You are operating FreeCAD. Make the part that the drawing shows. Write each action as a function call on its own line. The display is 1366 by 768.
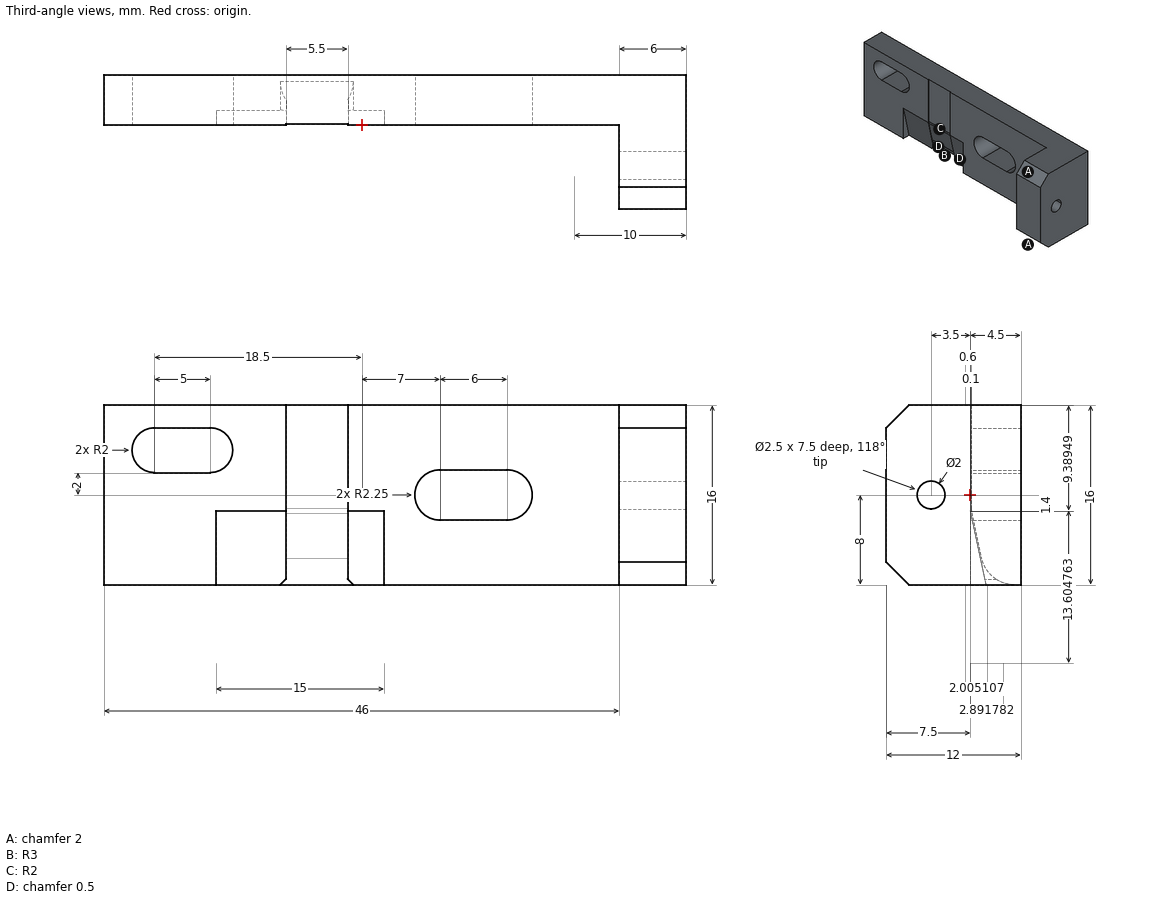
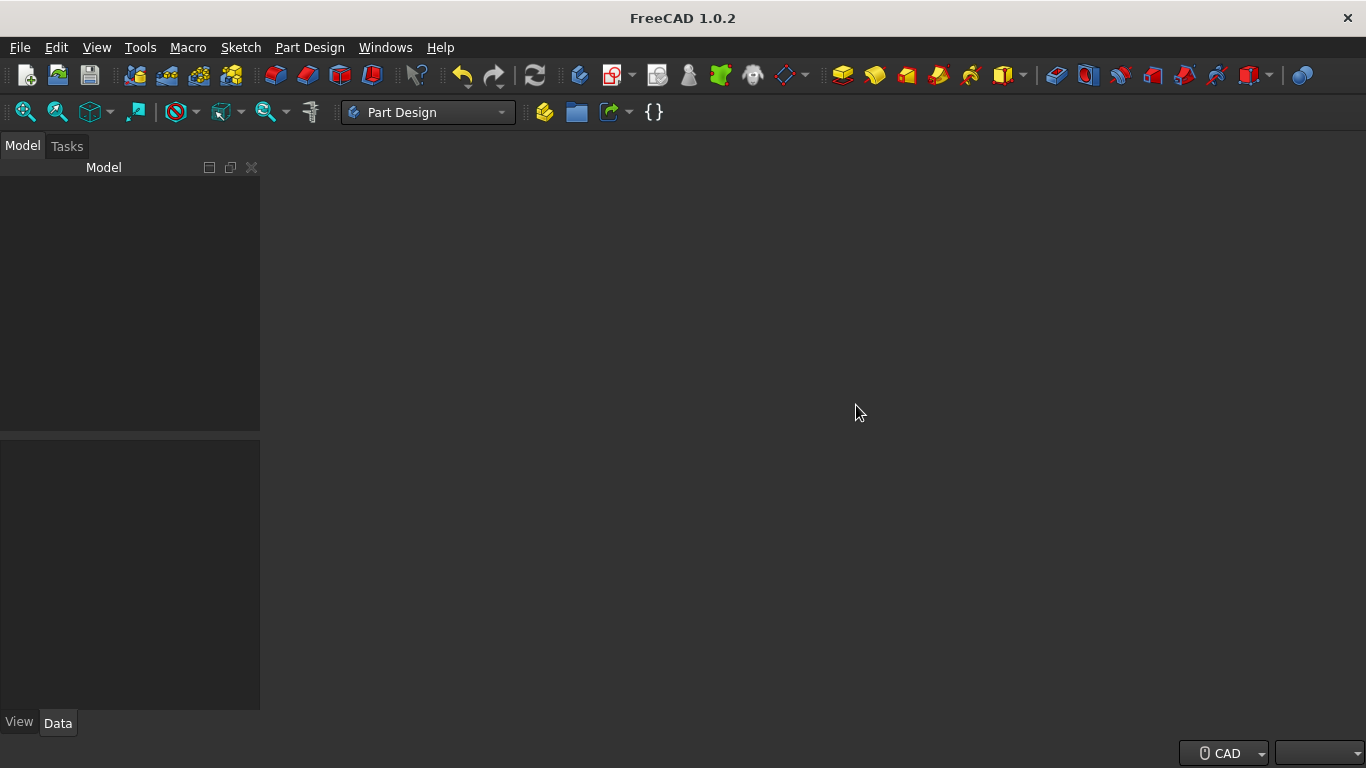
click(26, 76)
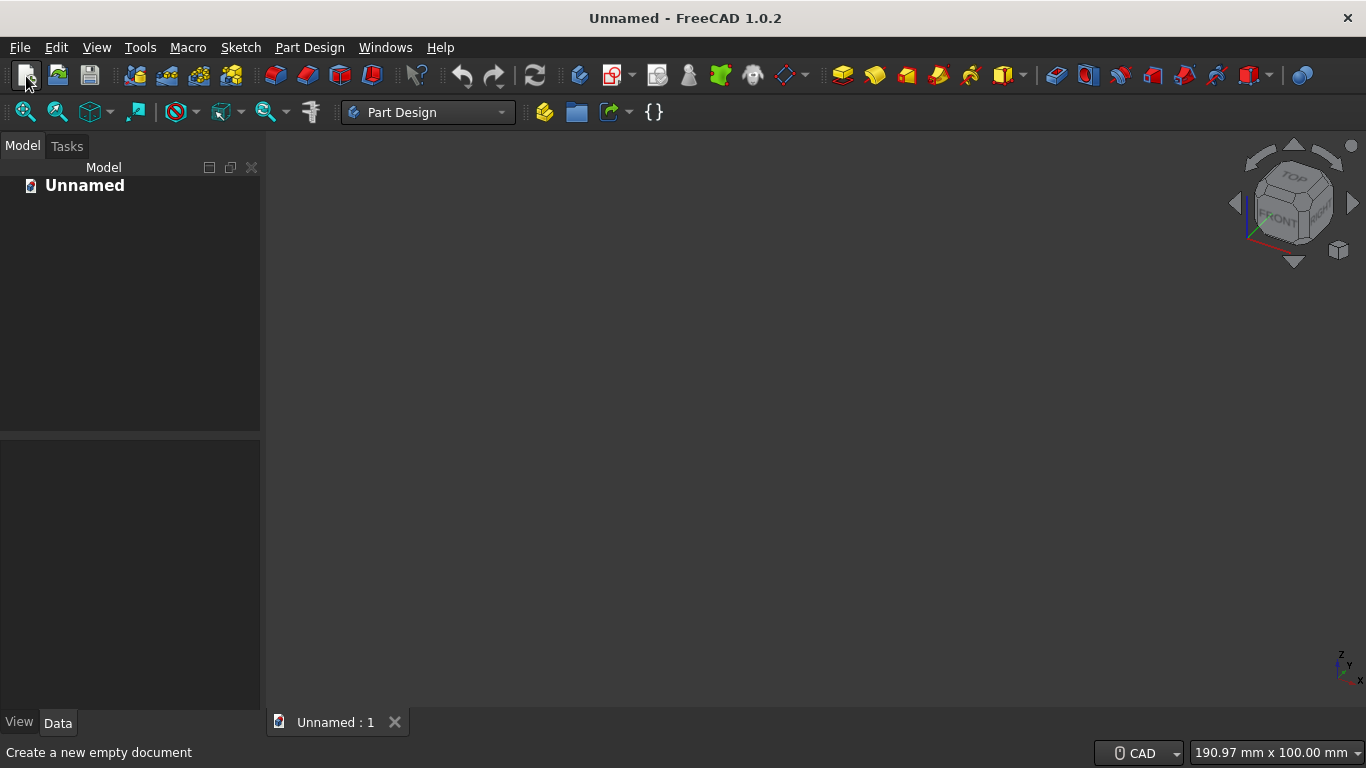
click(612, 76)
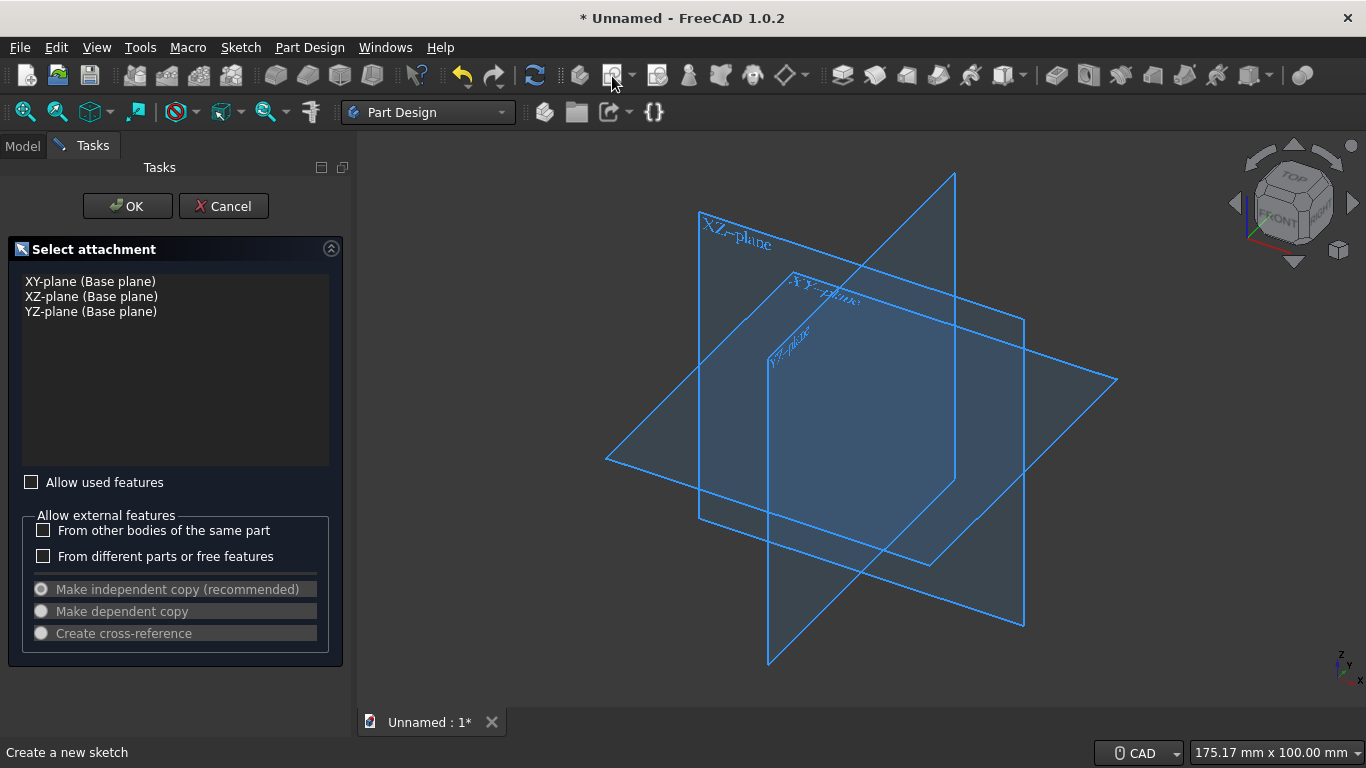
click(82, 296)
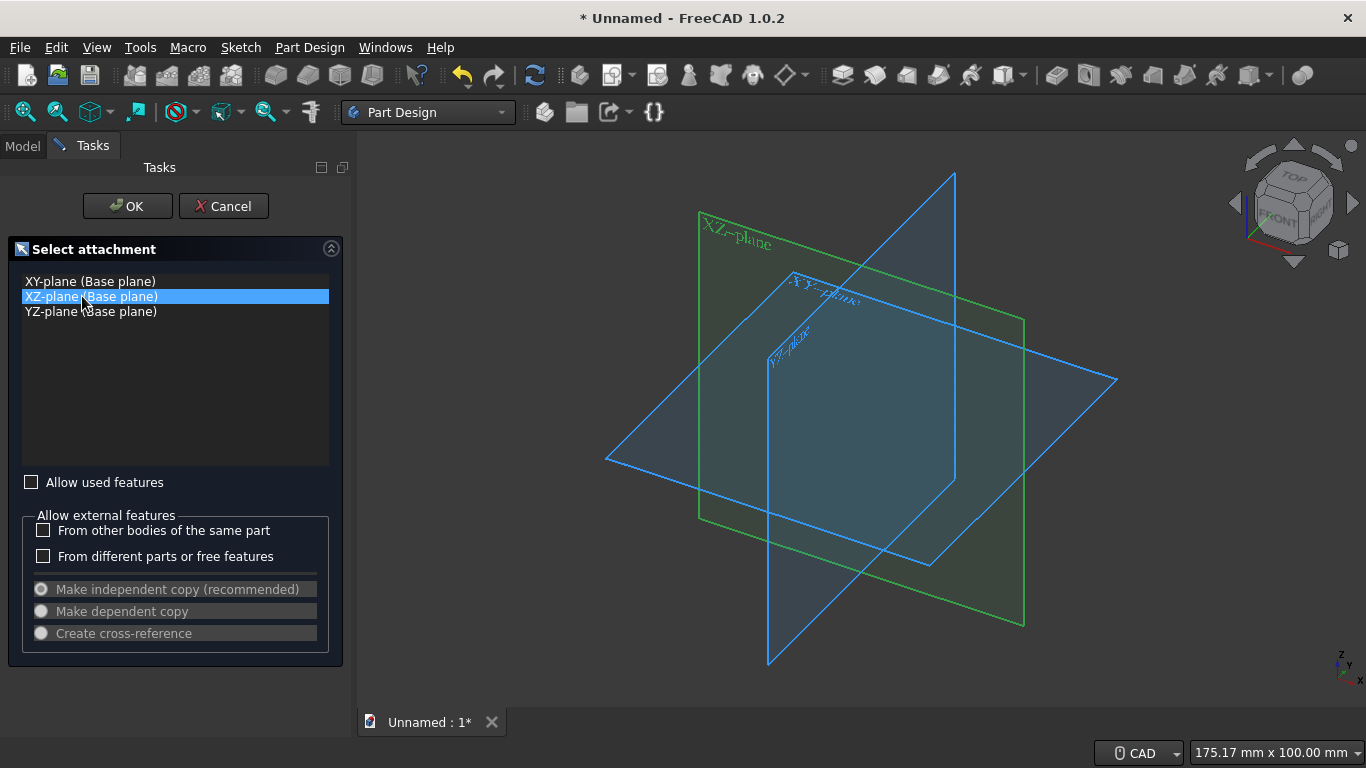
click(128, 206)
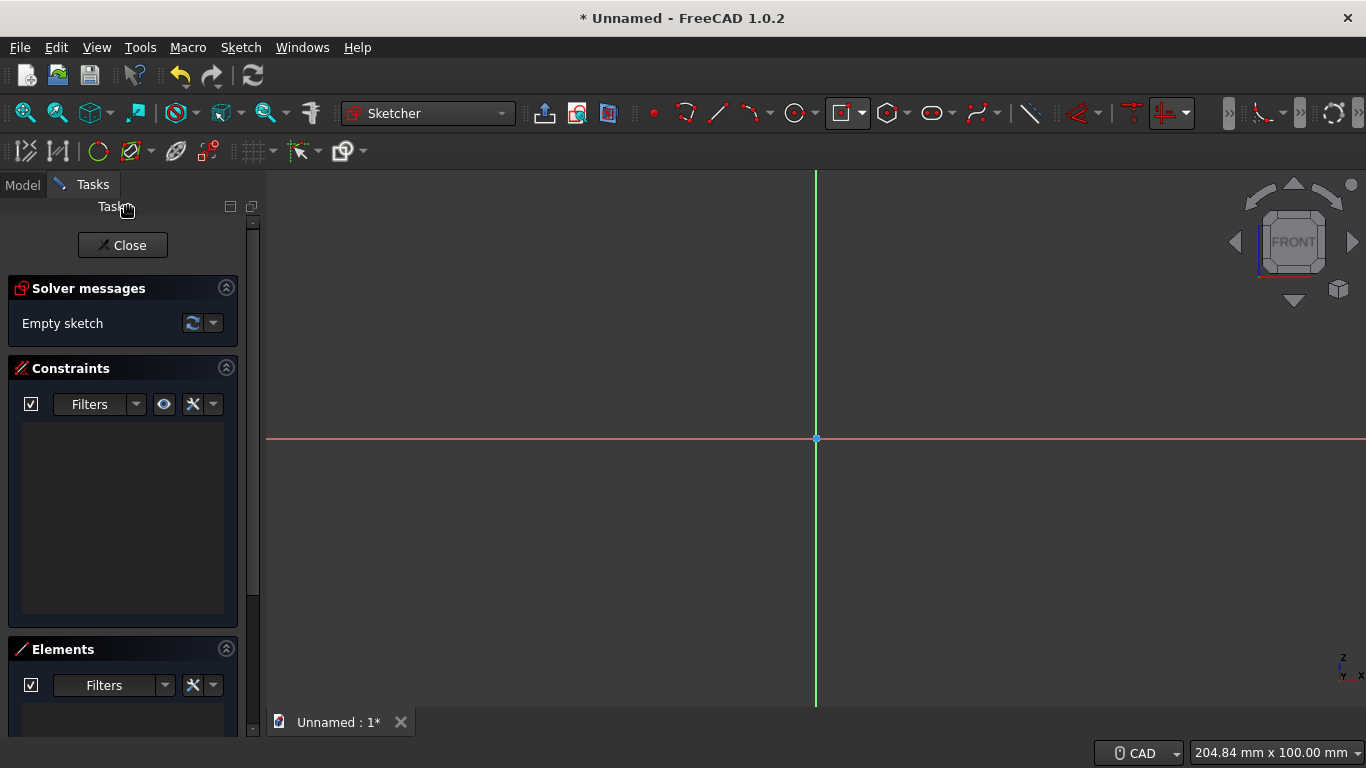
scroll(856, 439, up, 5)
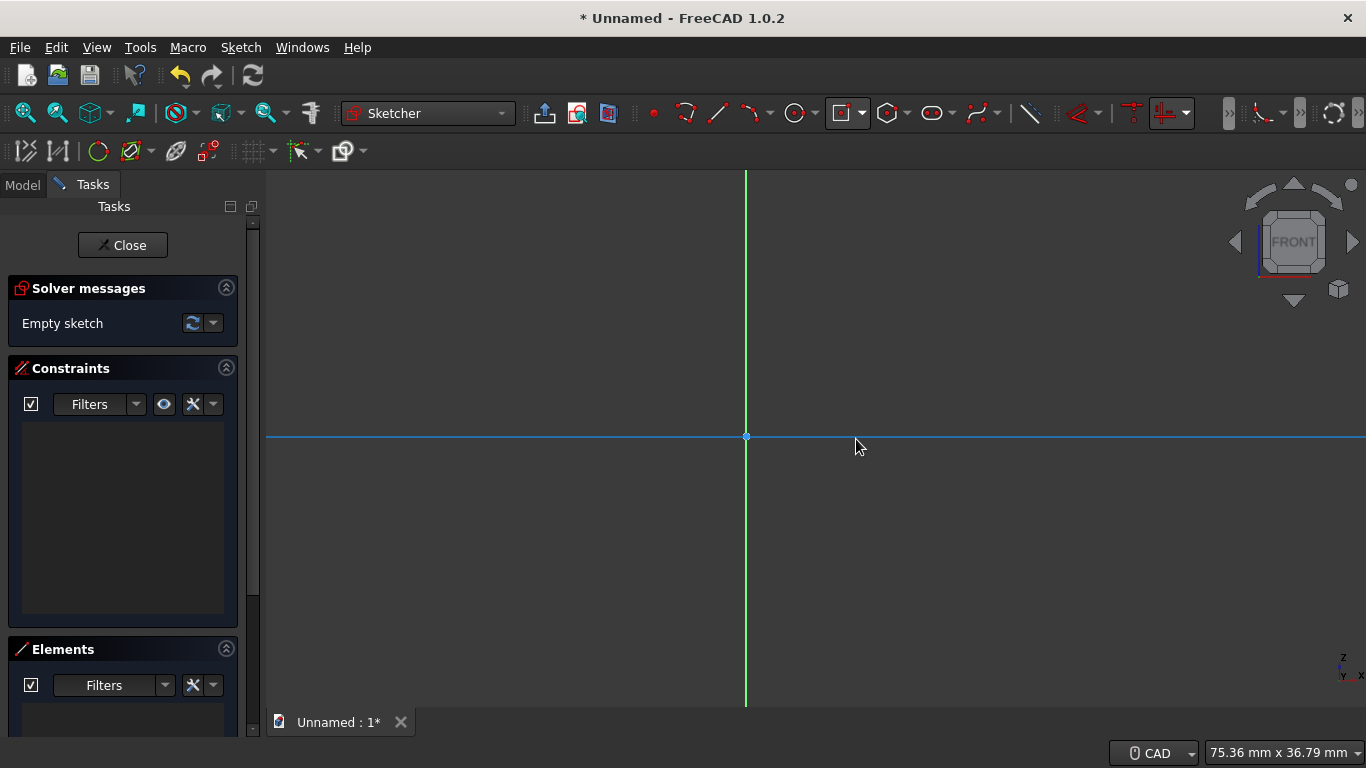
key(g)
key(v)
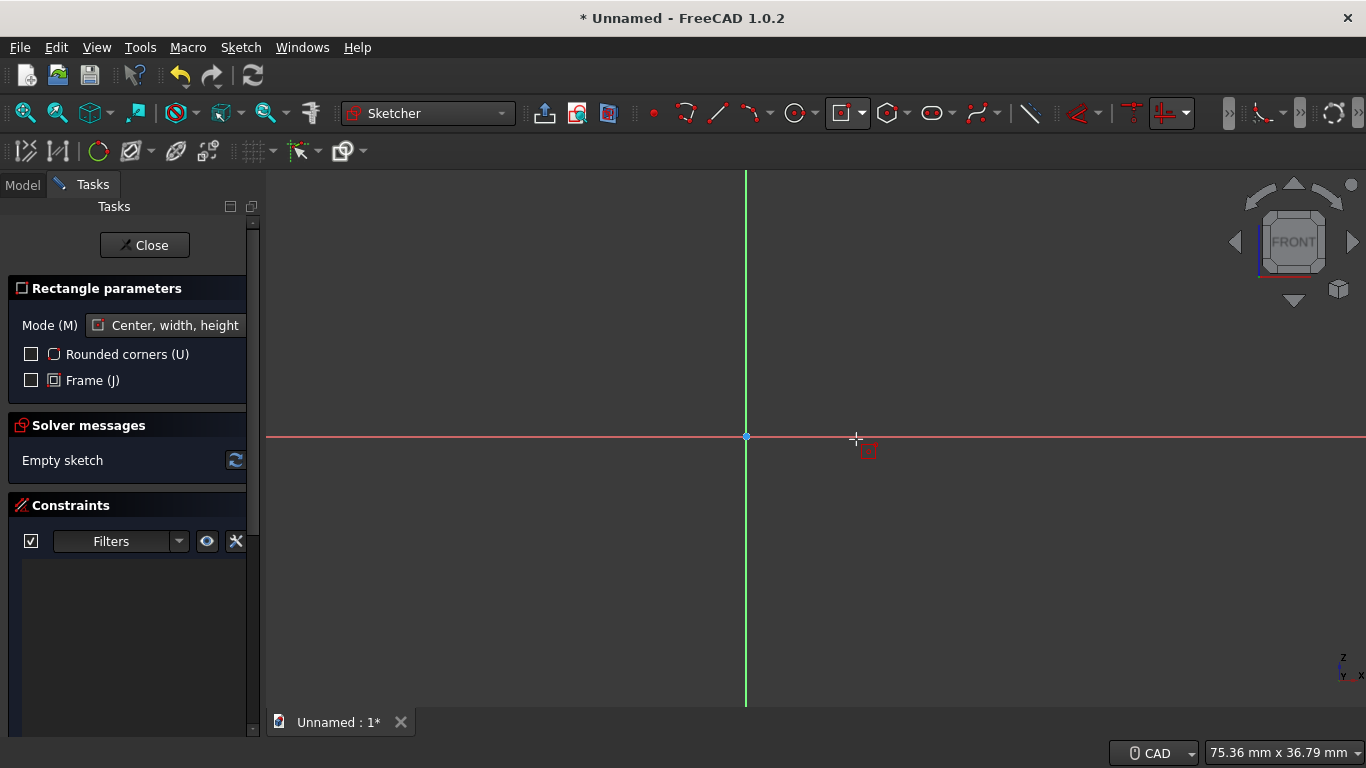
click(746, 437)
click(1082, 320)
key(Escape)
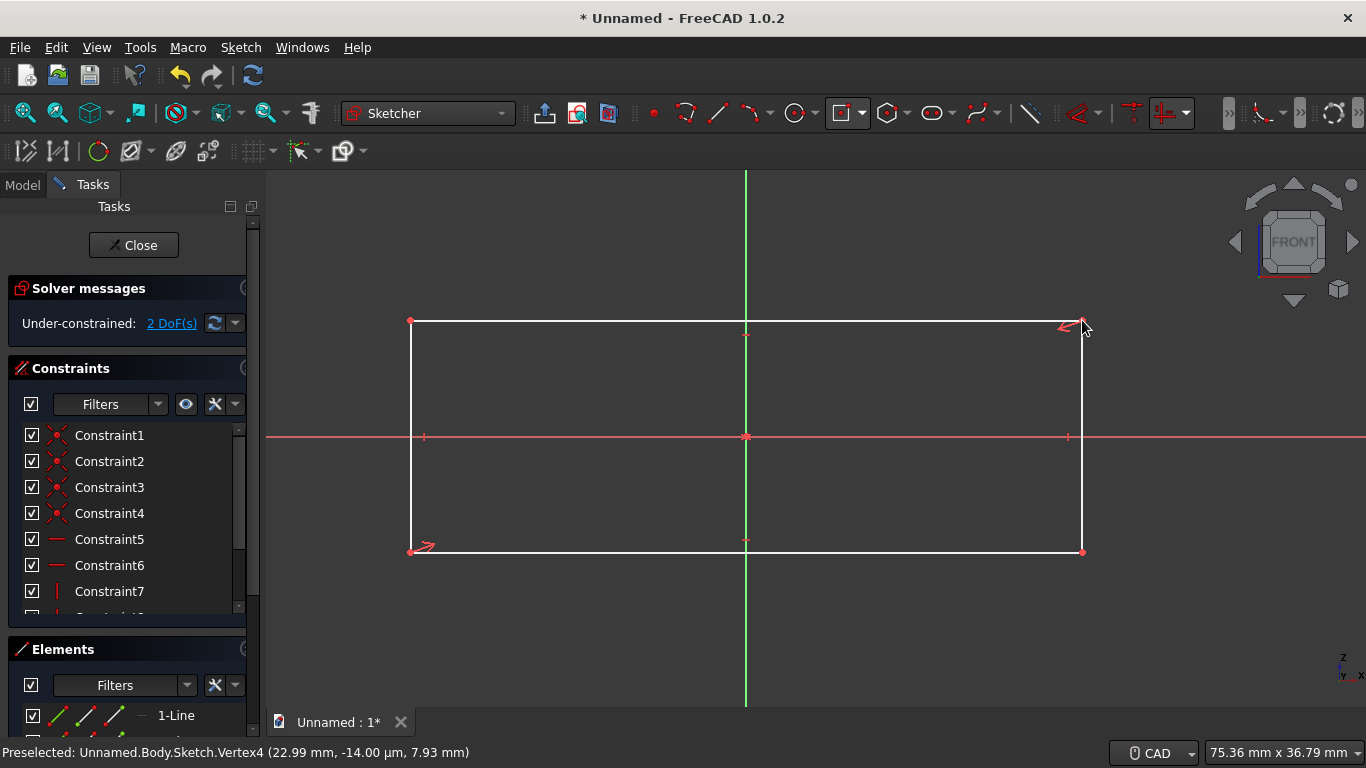
click(1078, 114)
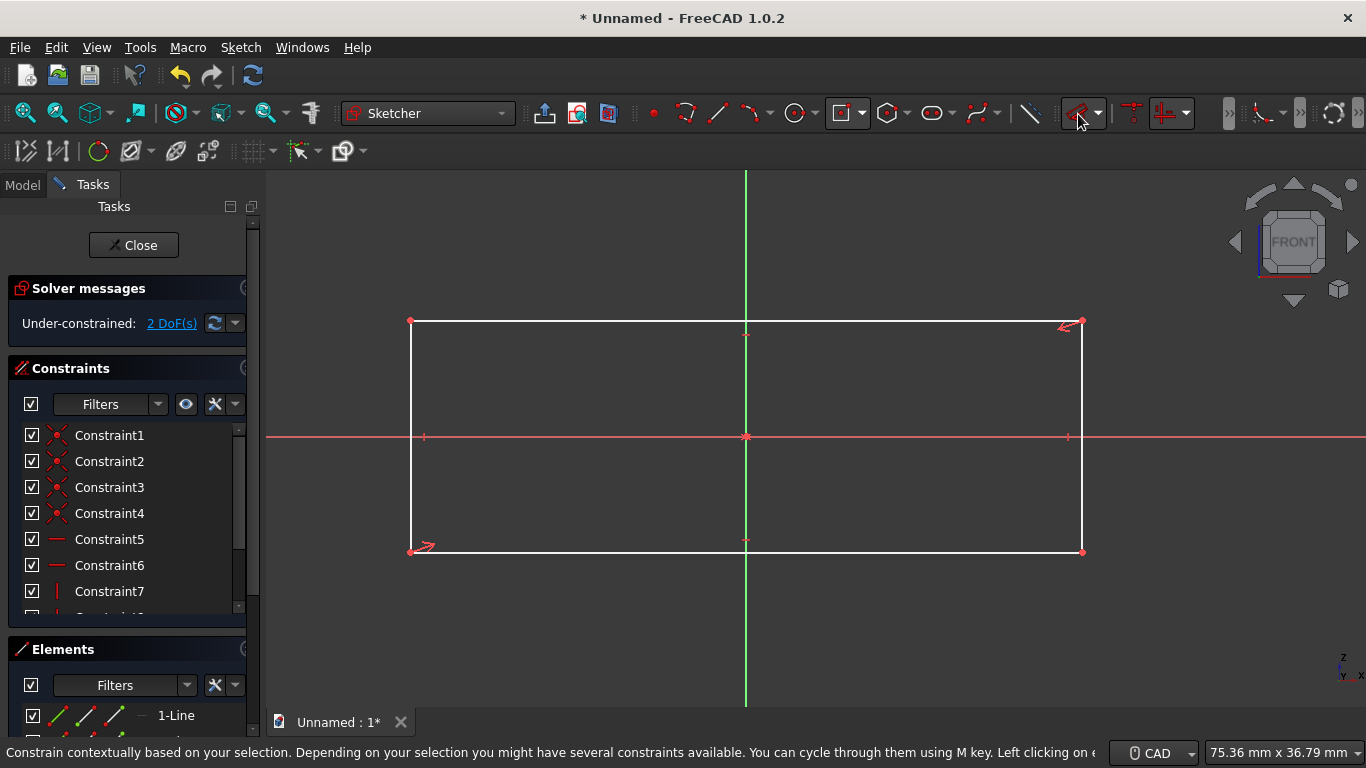
click(612, 553)
click(592, 587)